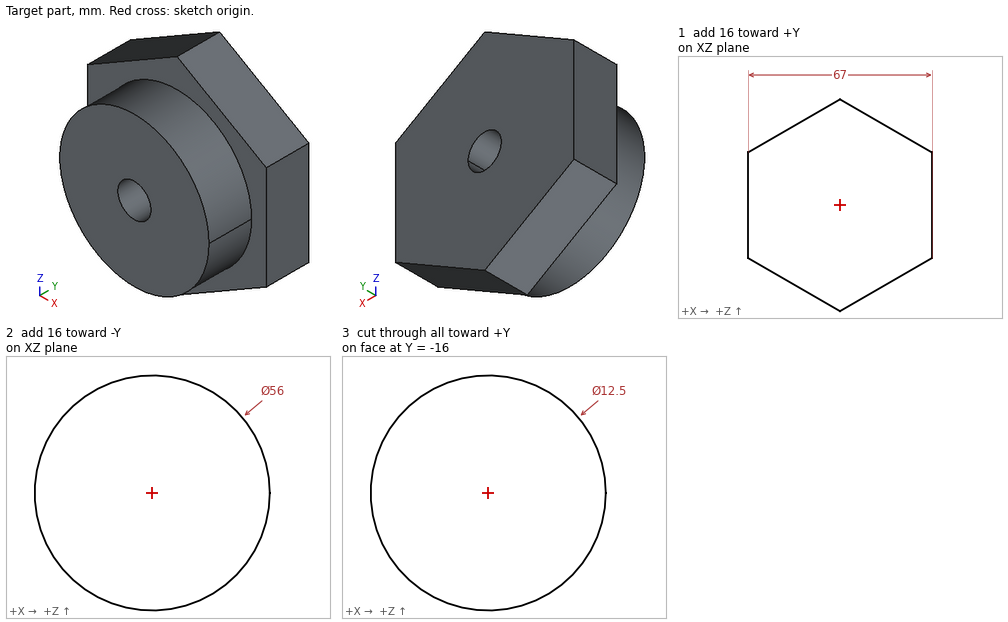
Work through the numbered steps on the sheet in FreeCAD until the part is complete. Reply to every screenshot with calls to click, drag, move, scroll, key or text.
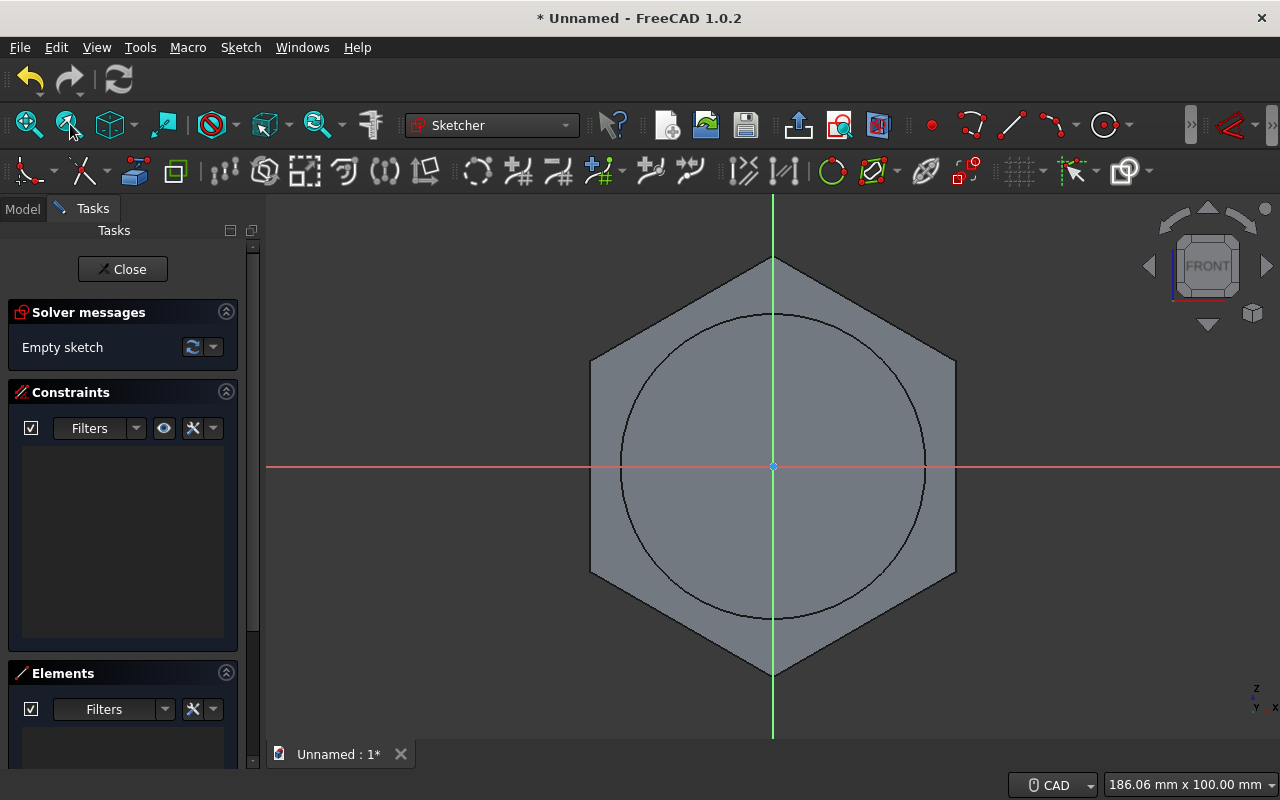
scroll(790, 466, up, 8)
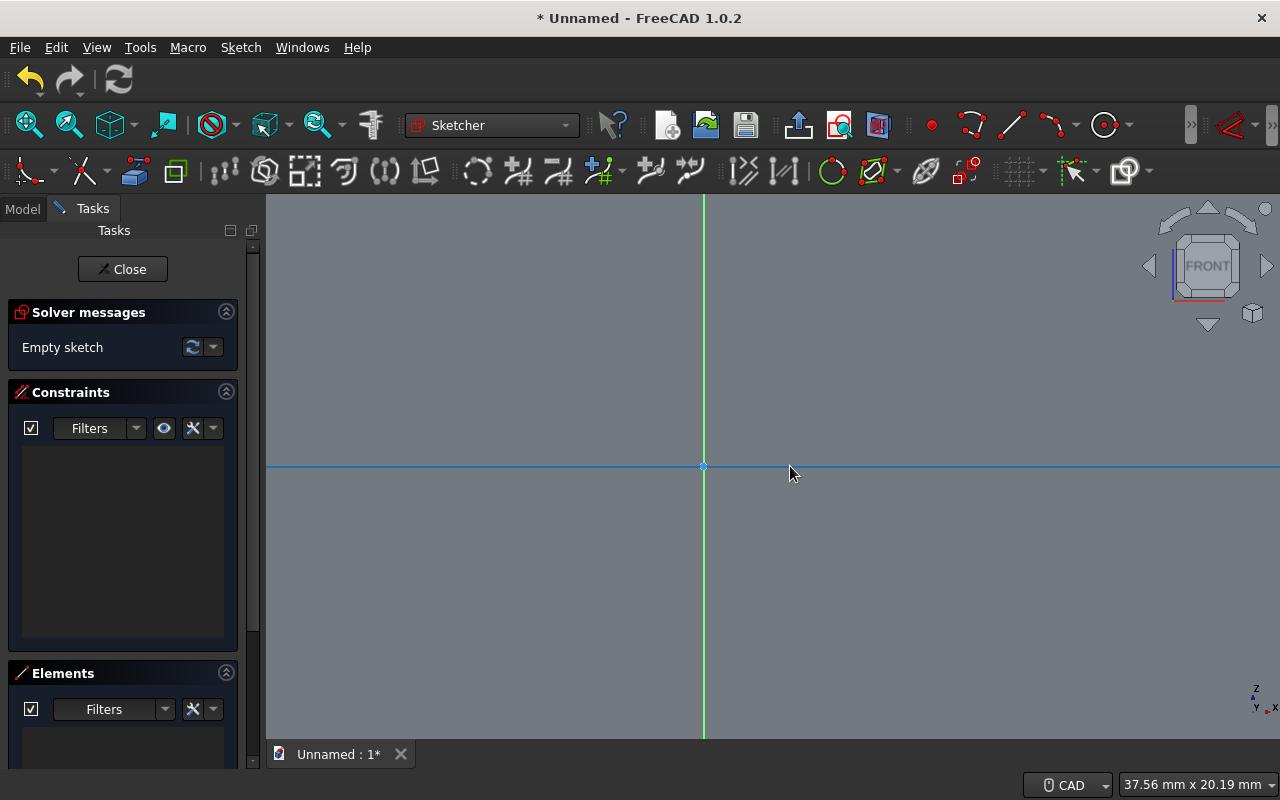
click(1106, 126)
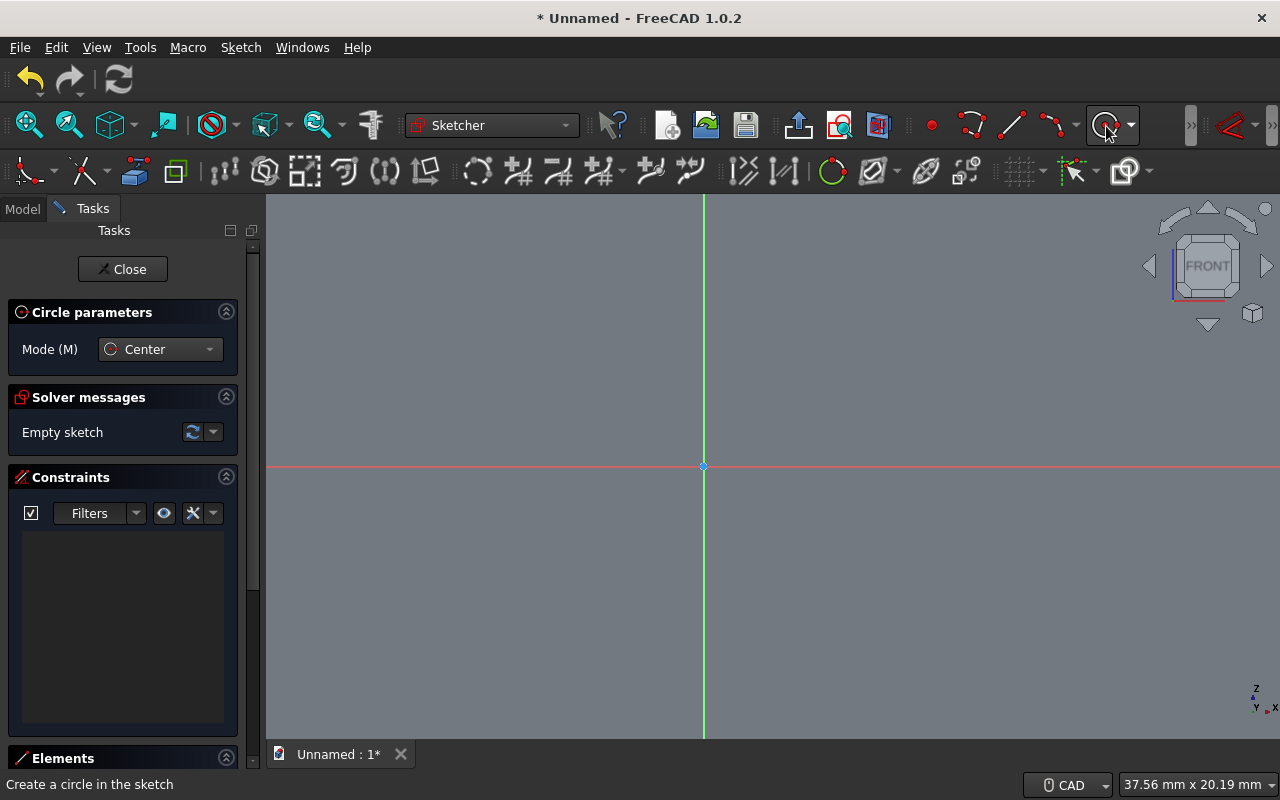
click(704, 466)
click(823, 347)
key(Escape)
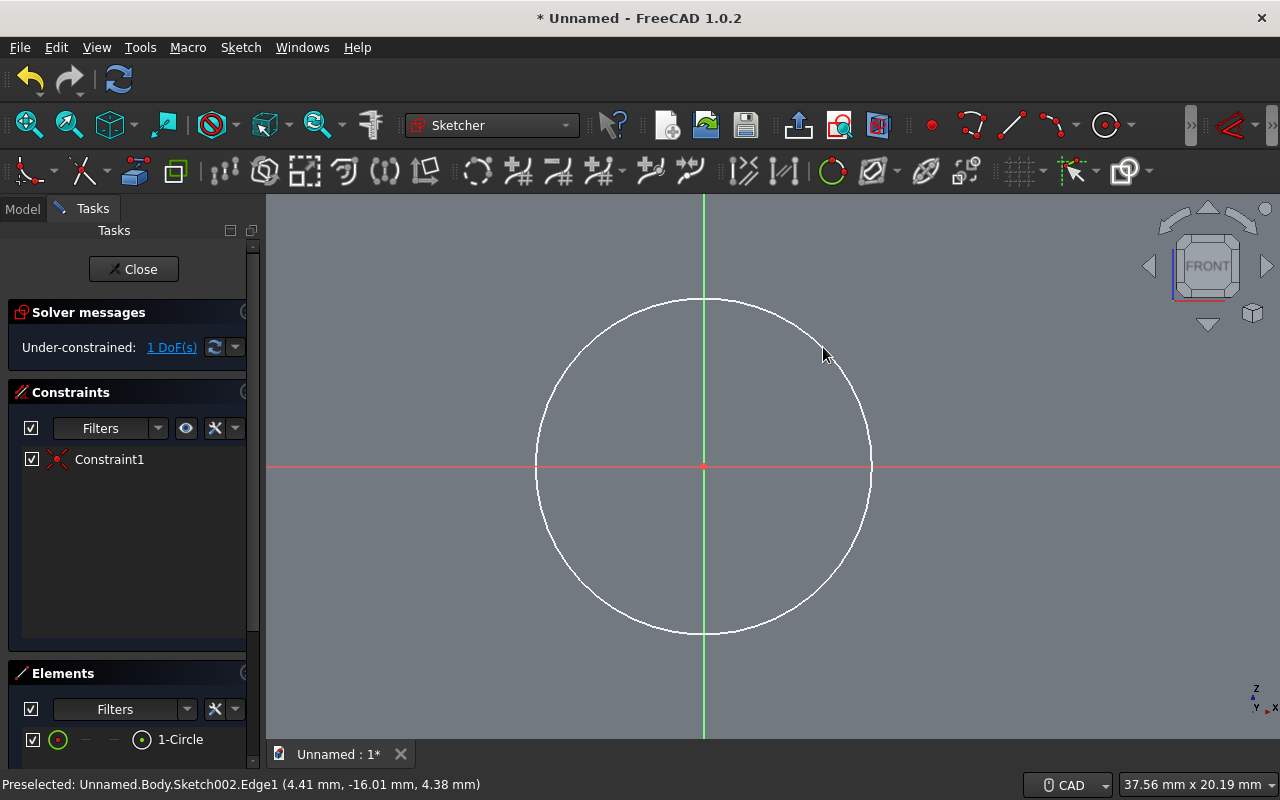
key(d)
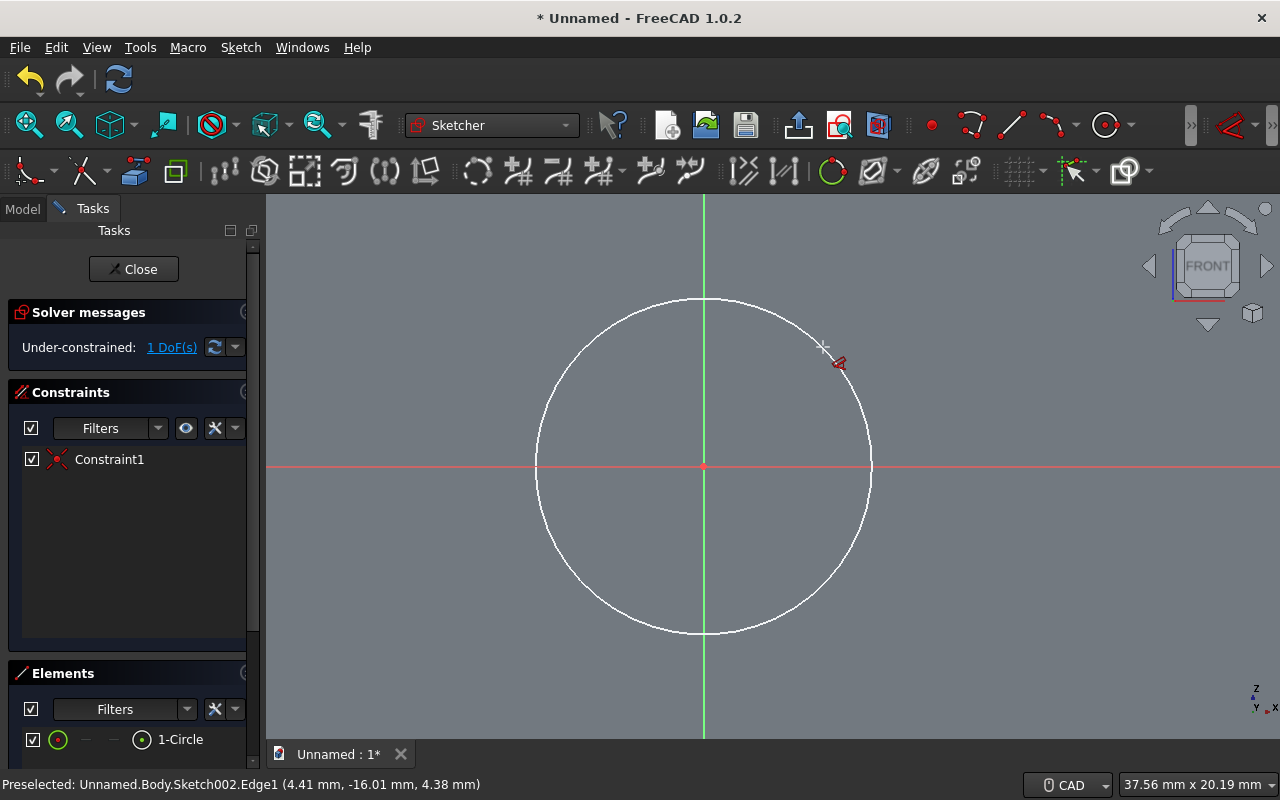
click(822, 347)
click(845, 324)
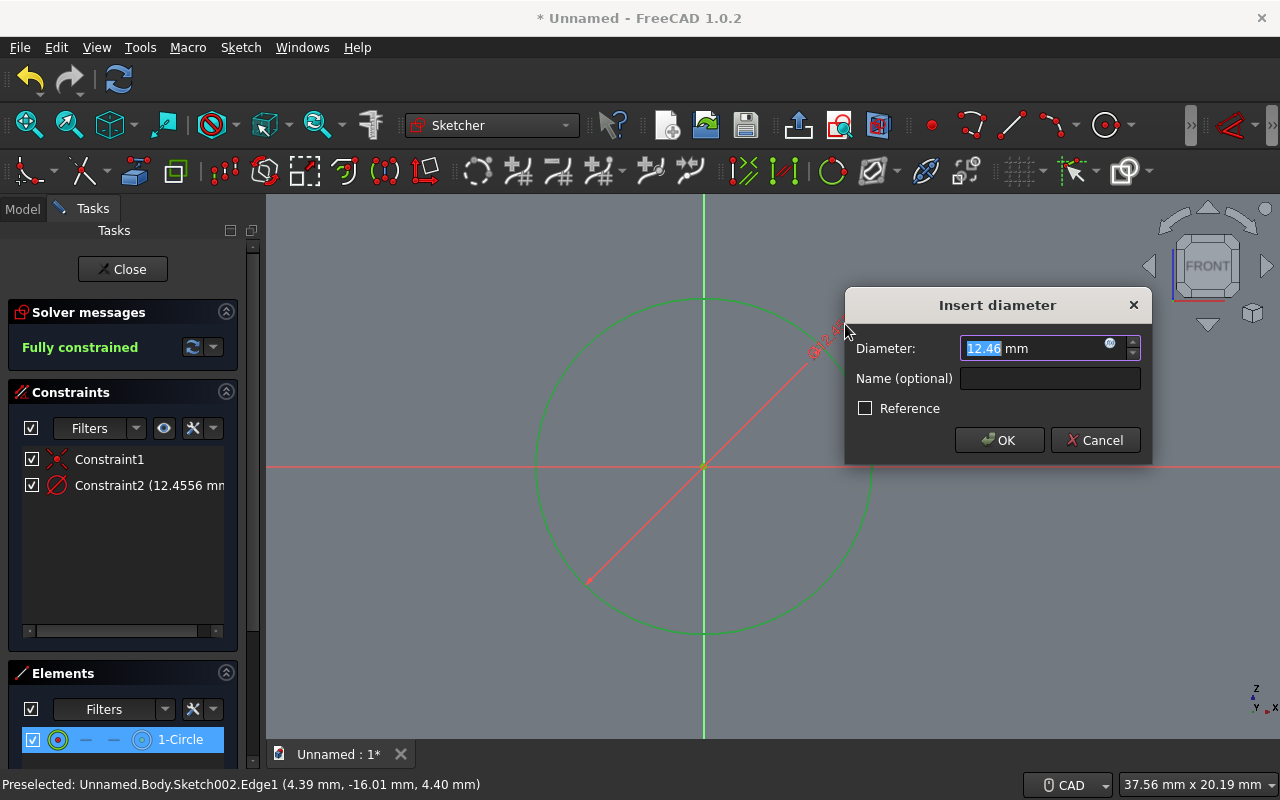
text(12.5)
key(Return)
key(Escape)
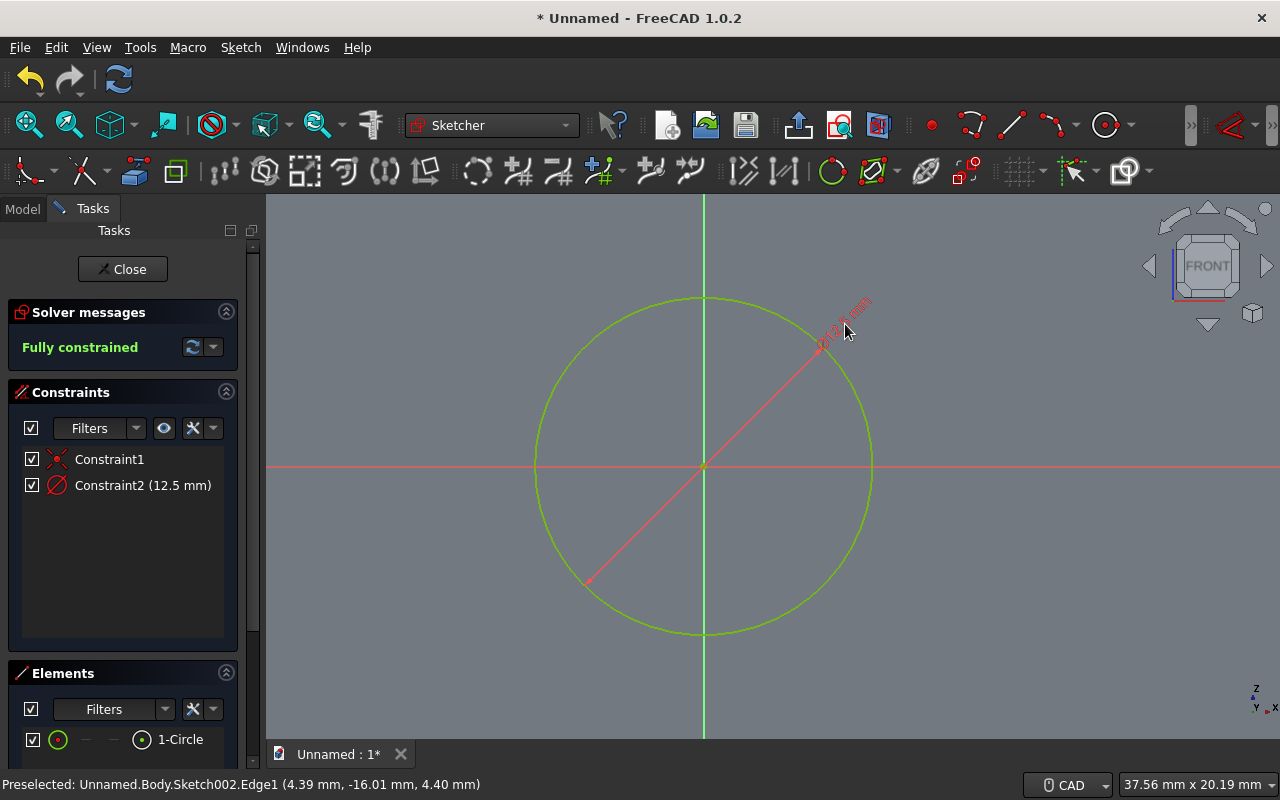
click(123, 269)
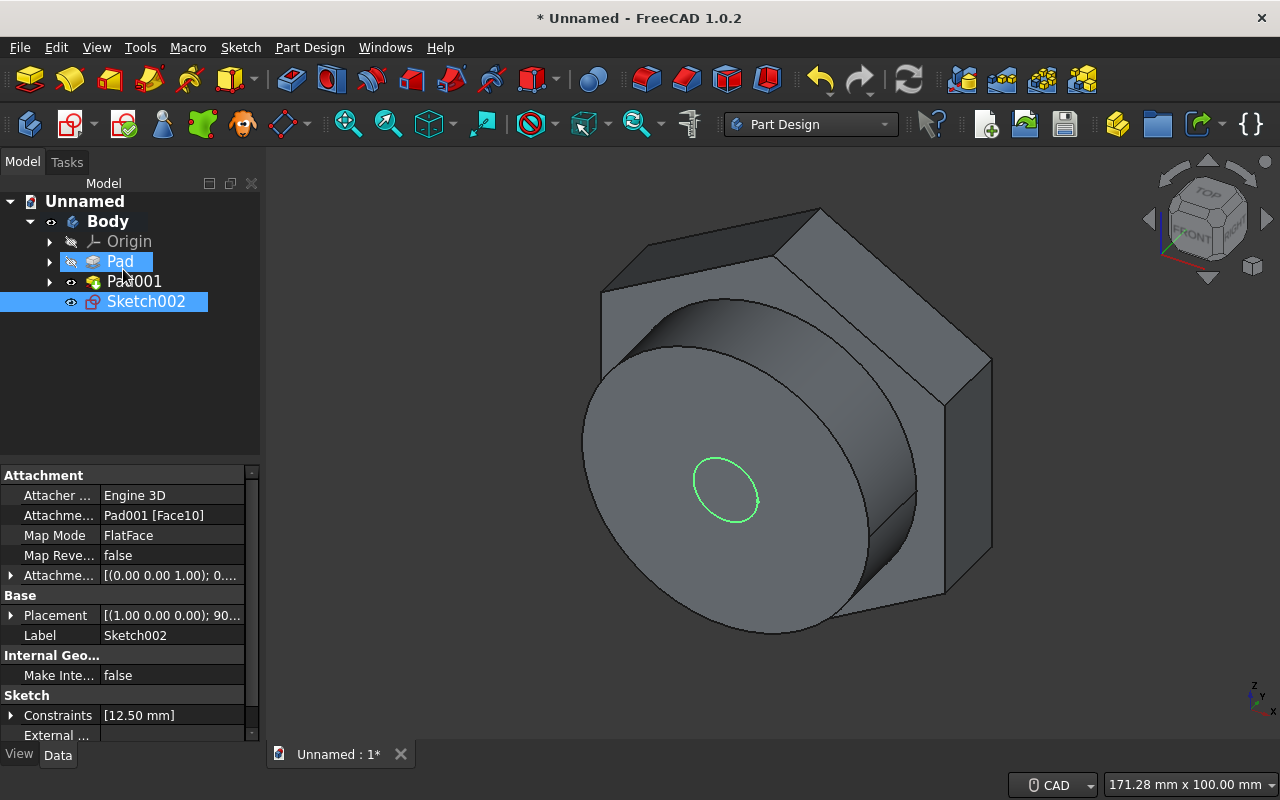
click(292, 80)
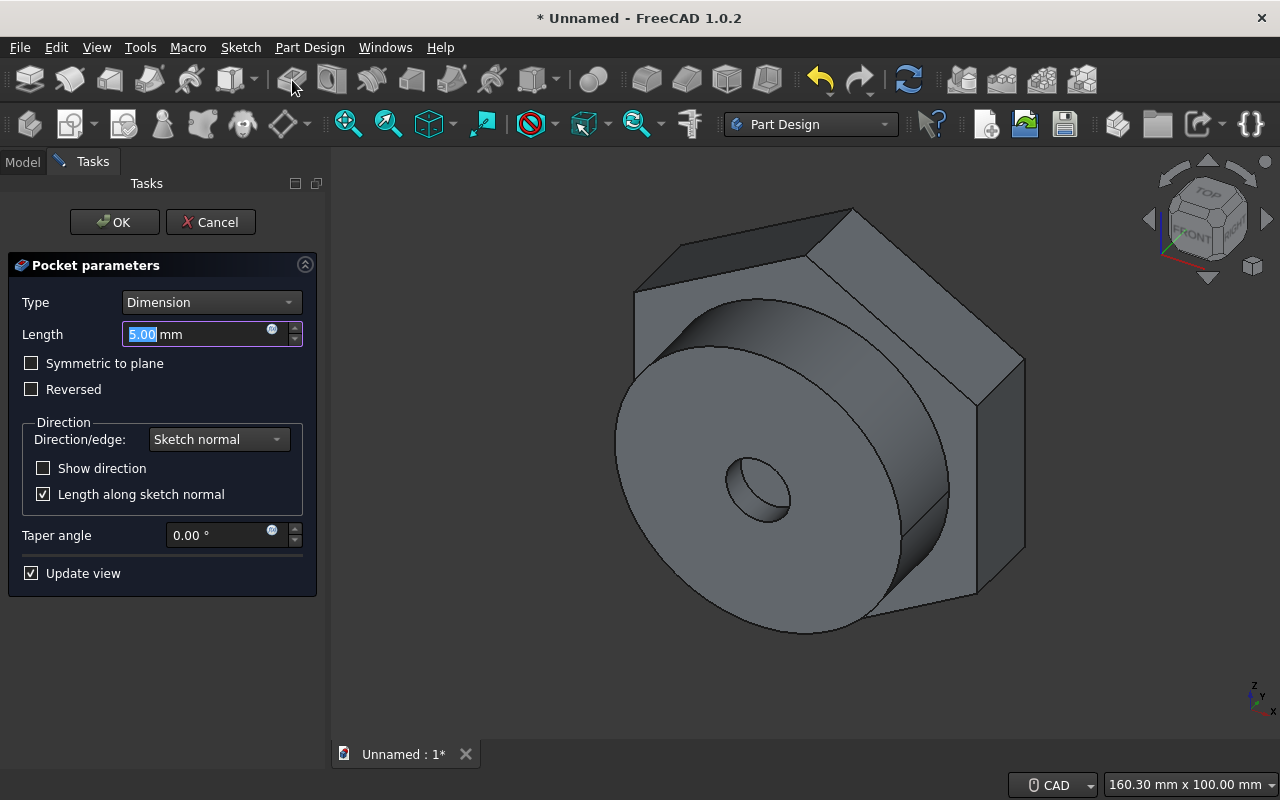
click(212, 302)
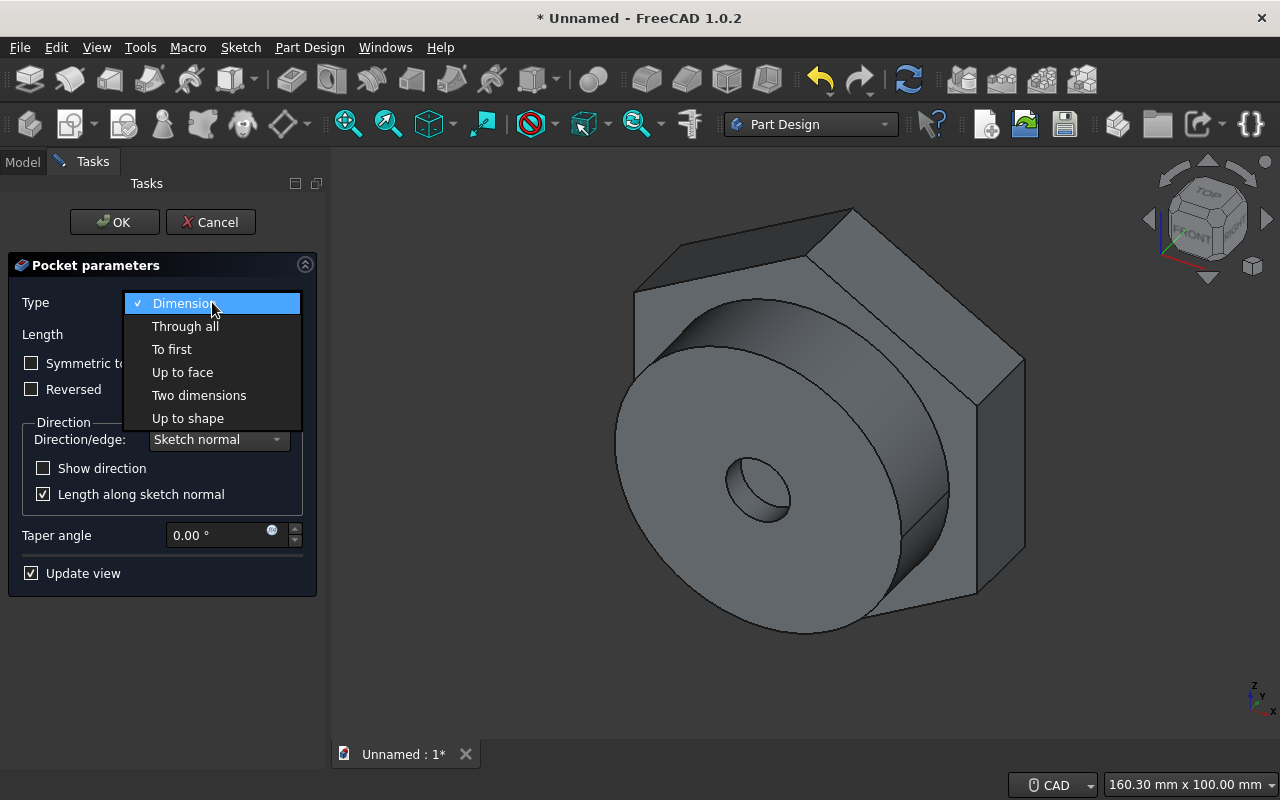
click(212, 326)